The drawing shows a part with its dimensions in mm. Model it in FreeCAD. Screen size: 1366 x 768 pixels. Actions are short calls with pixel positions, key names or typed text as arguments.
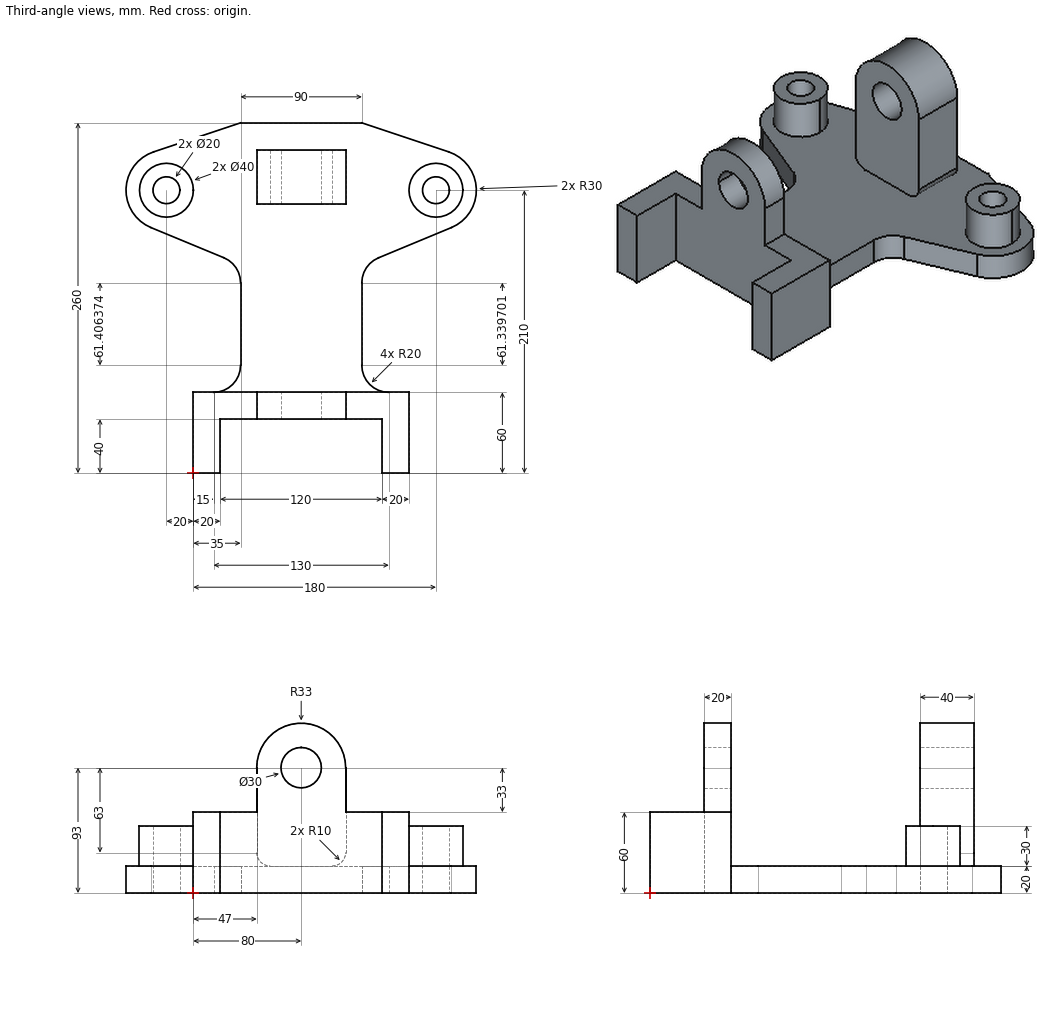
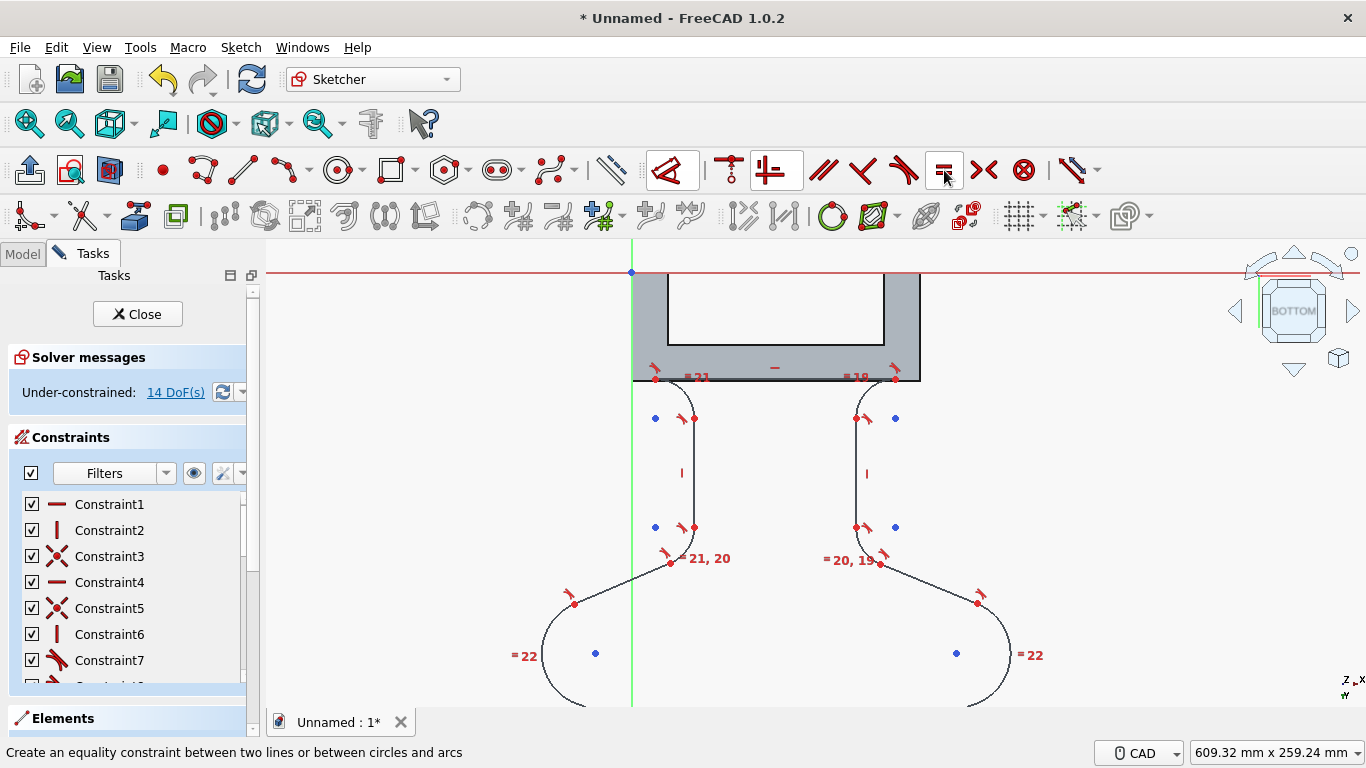
click(860, 400)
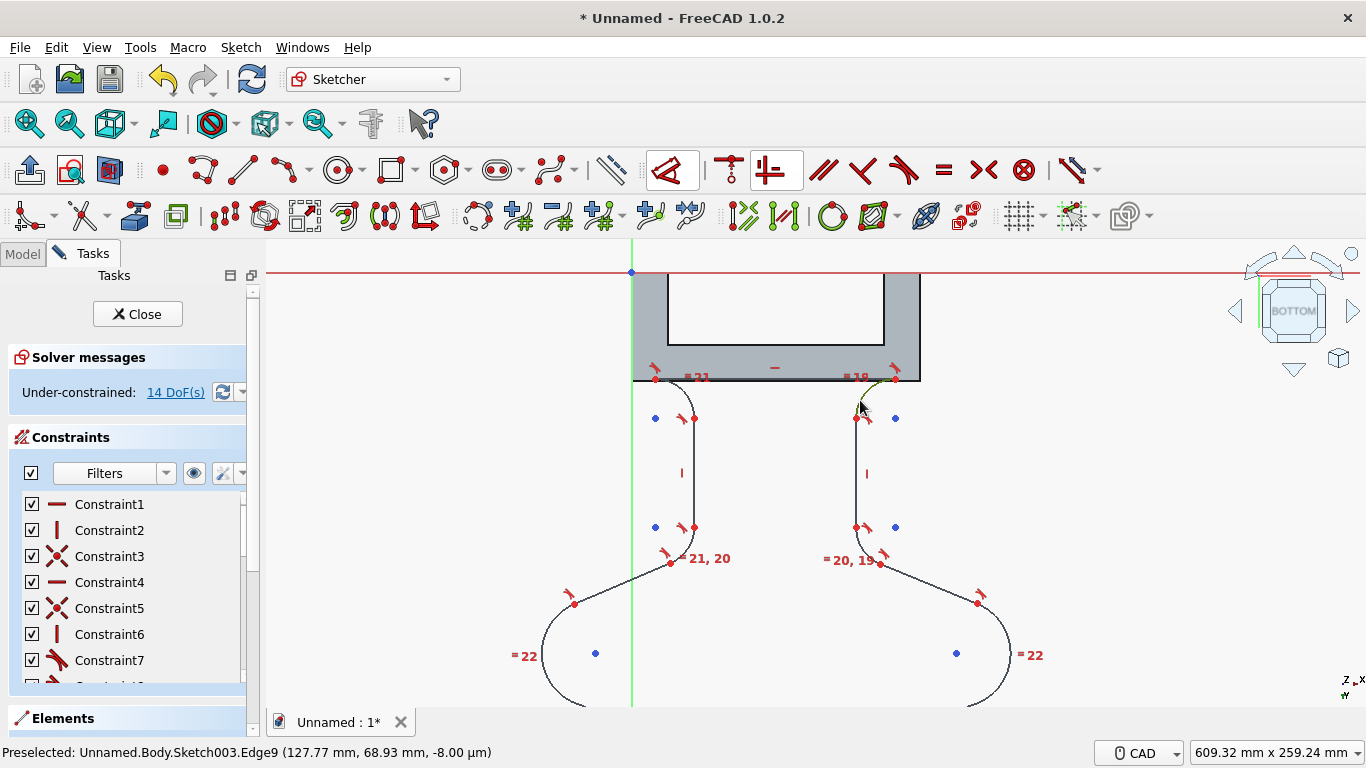
click(694, 170)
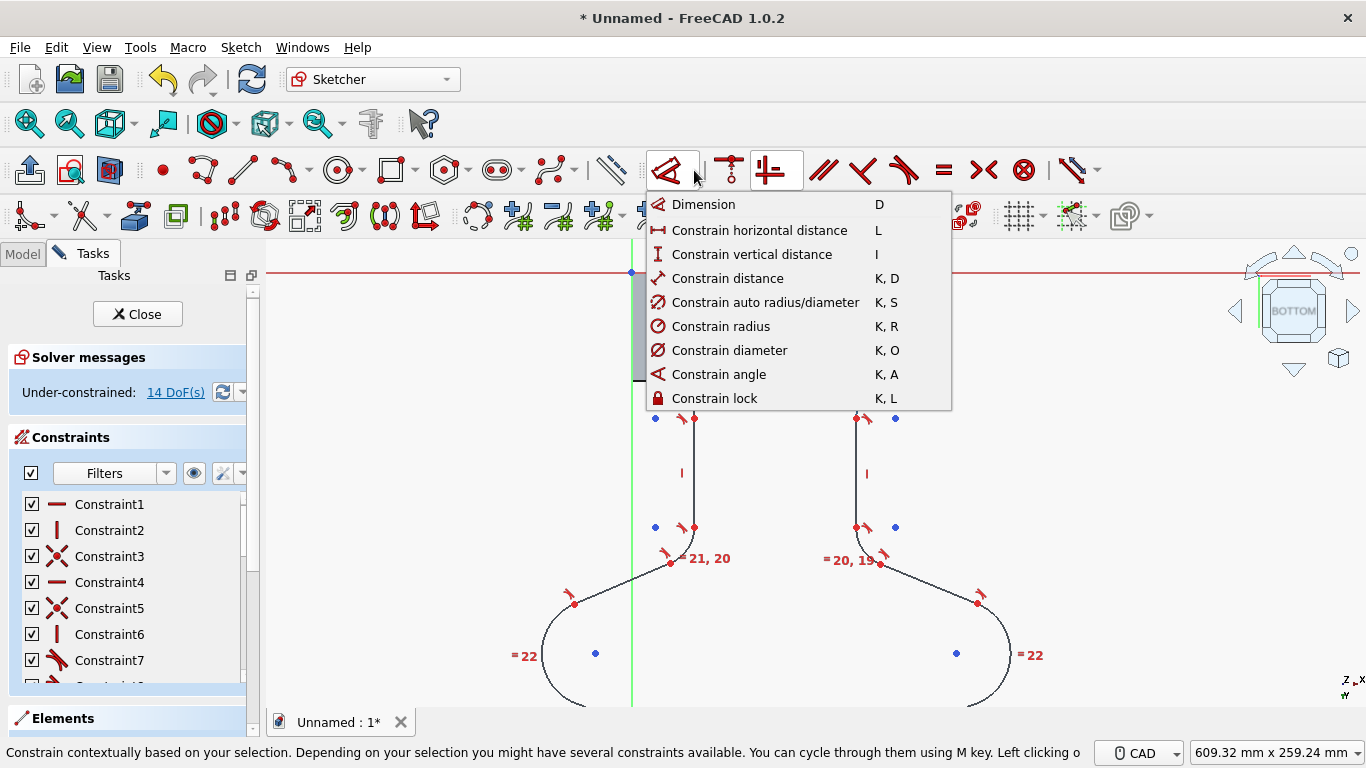
click(799, 326)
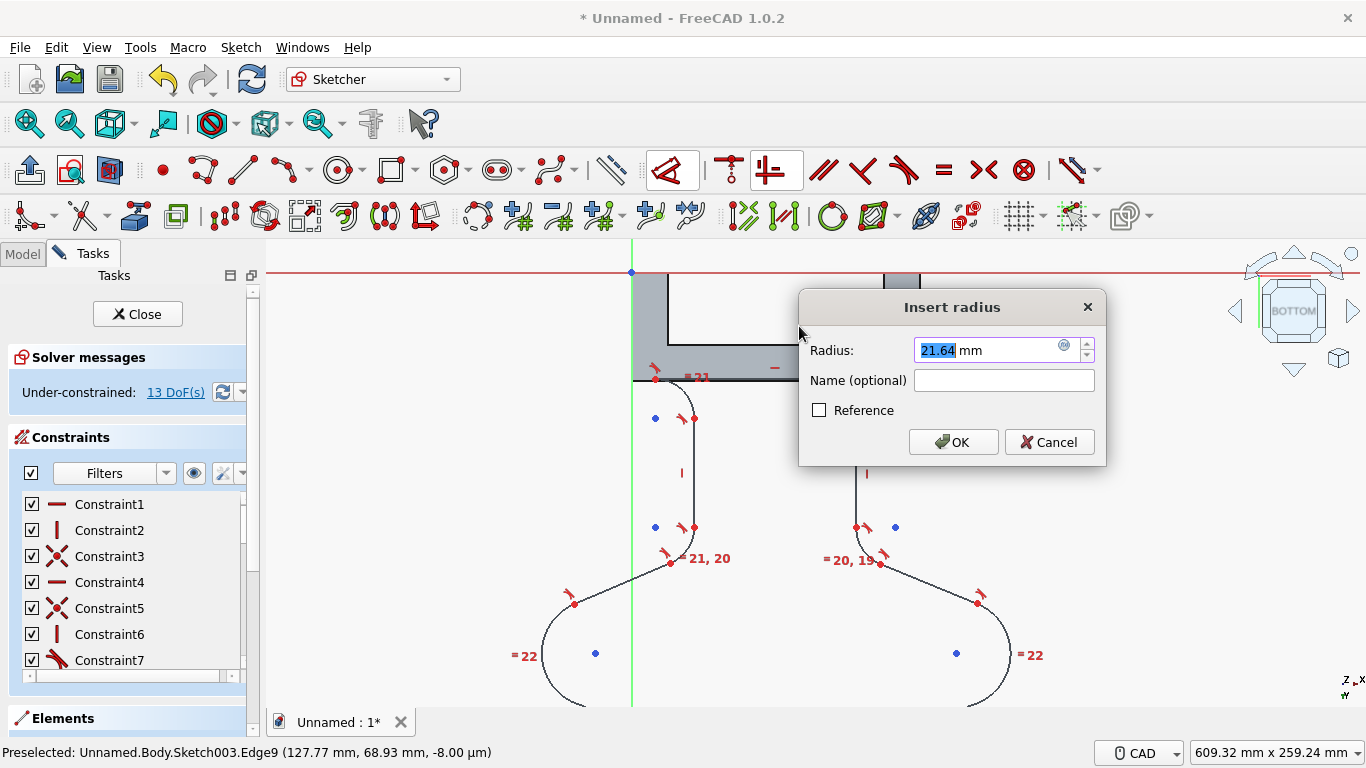
text(20)
key(Return)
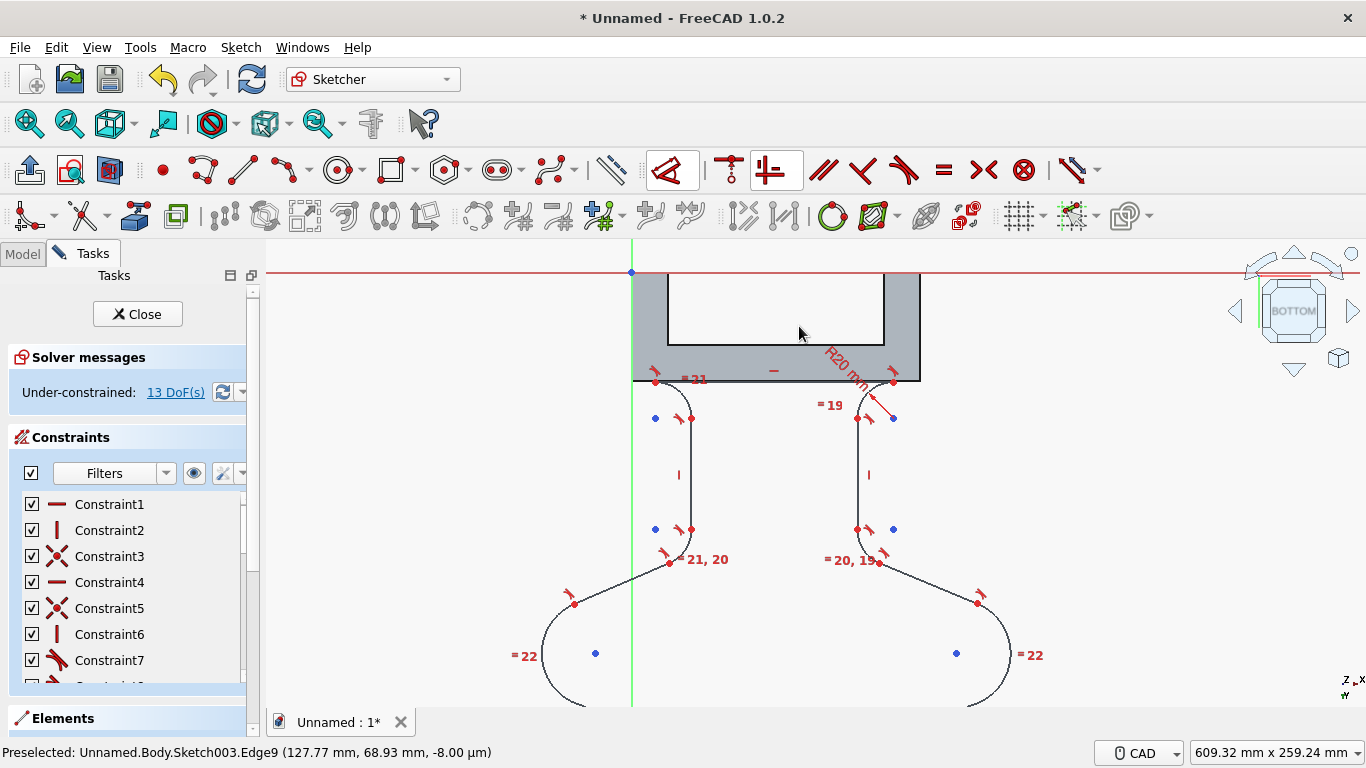
click(1005, 630)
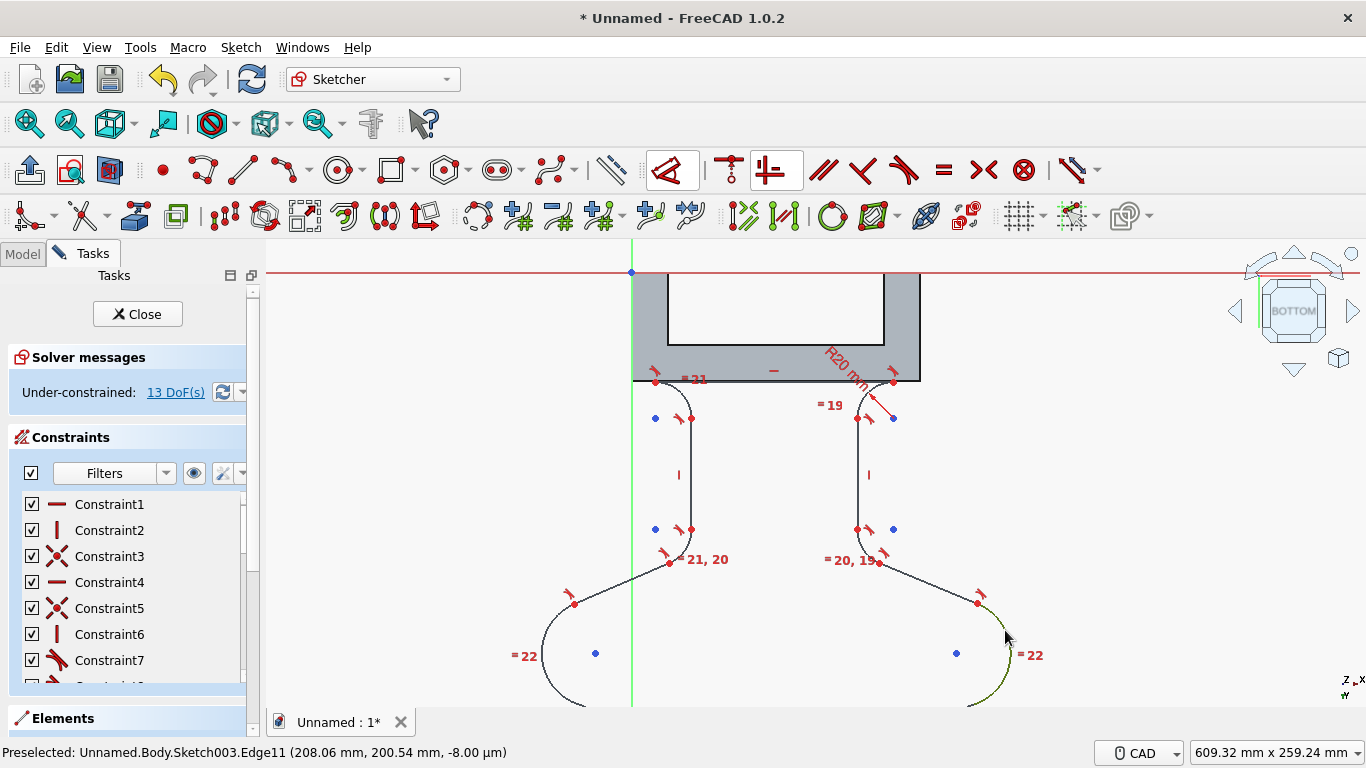
key(k)
key(r)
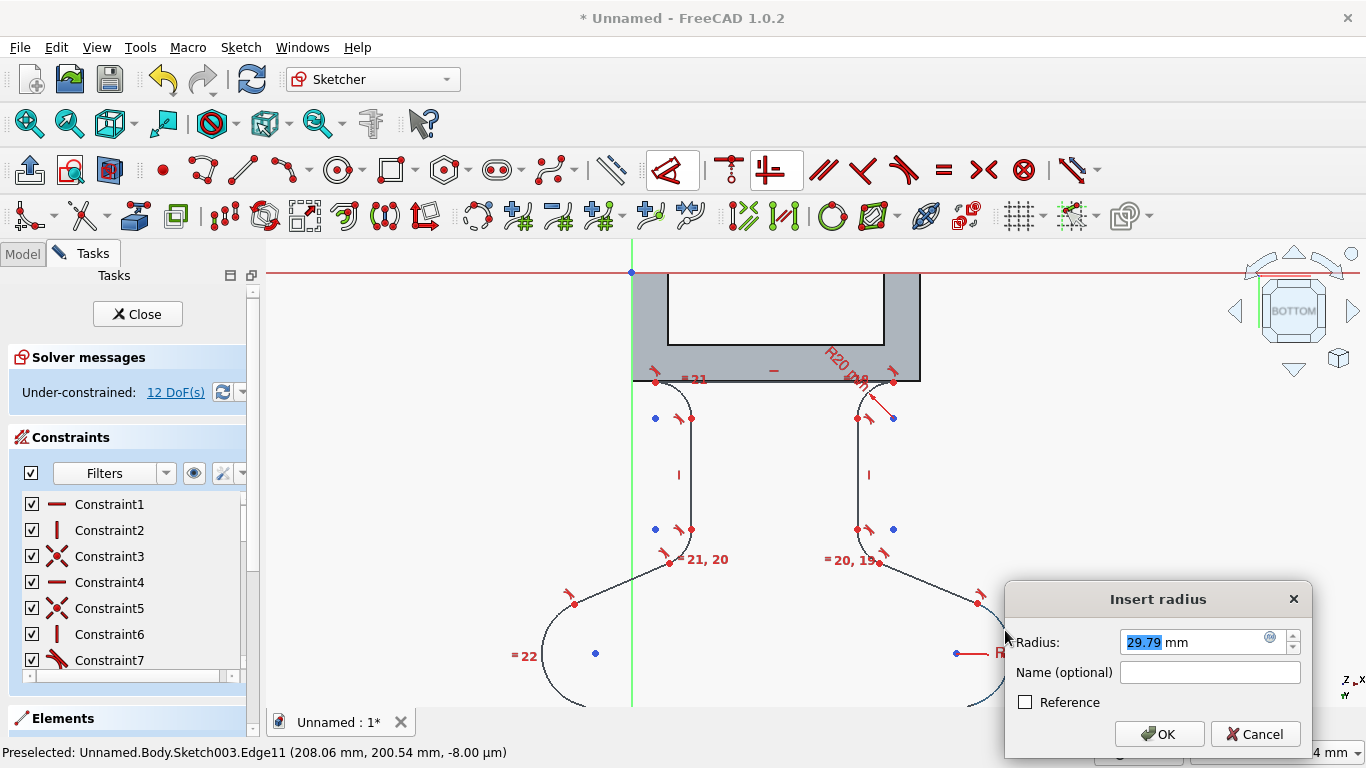
text(30)
key(Return)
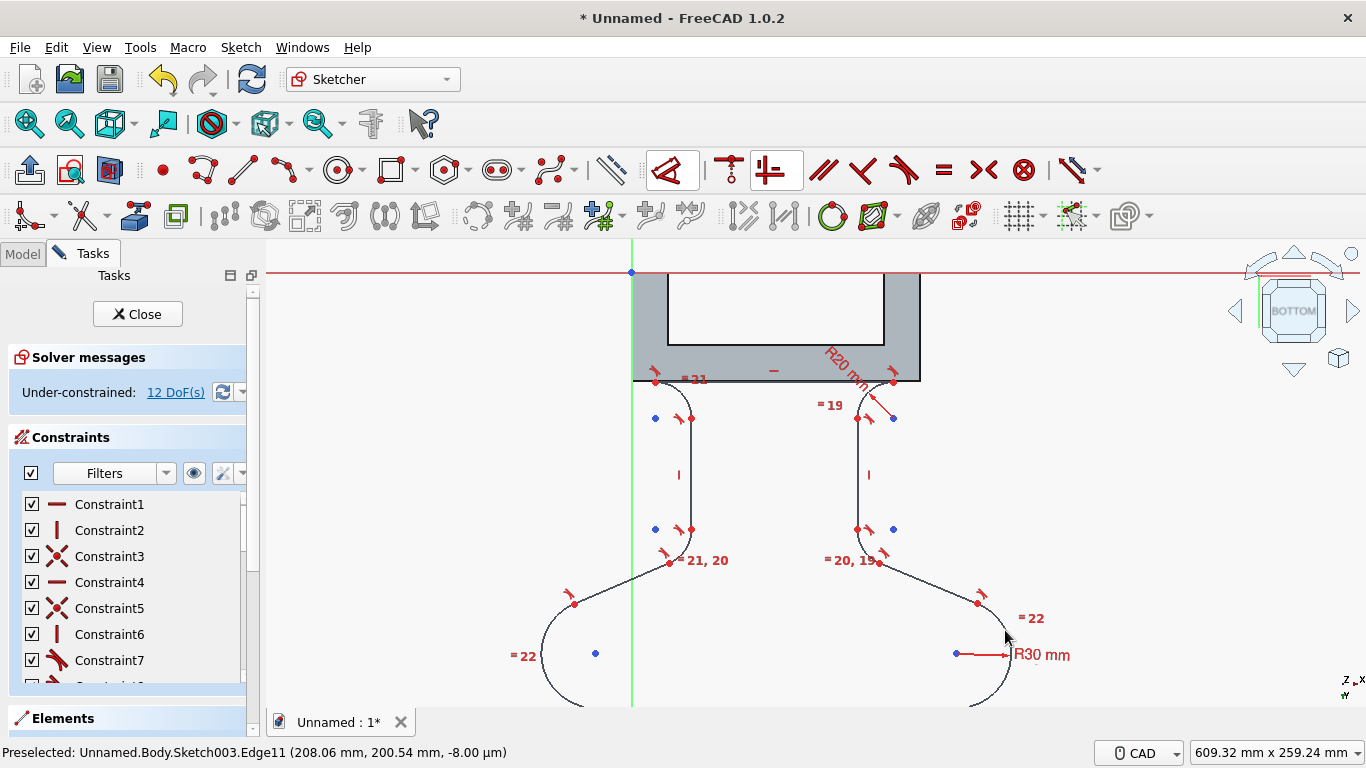
scroll(689, 403, down, 2)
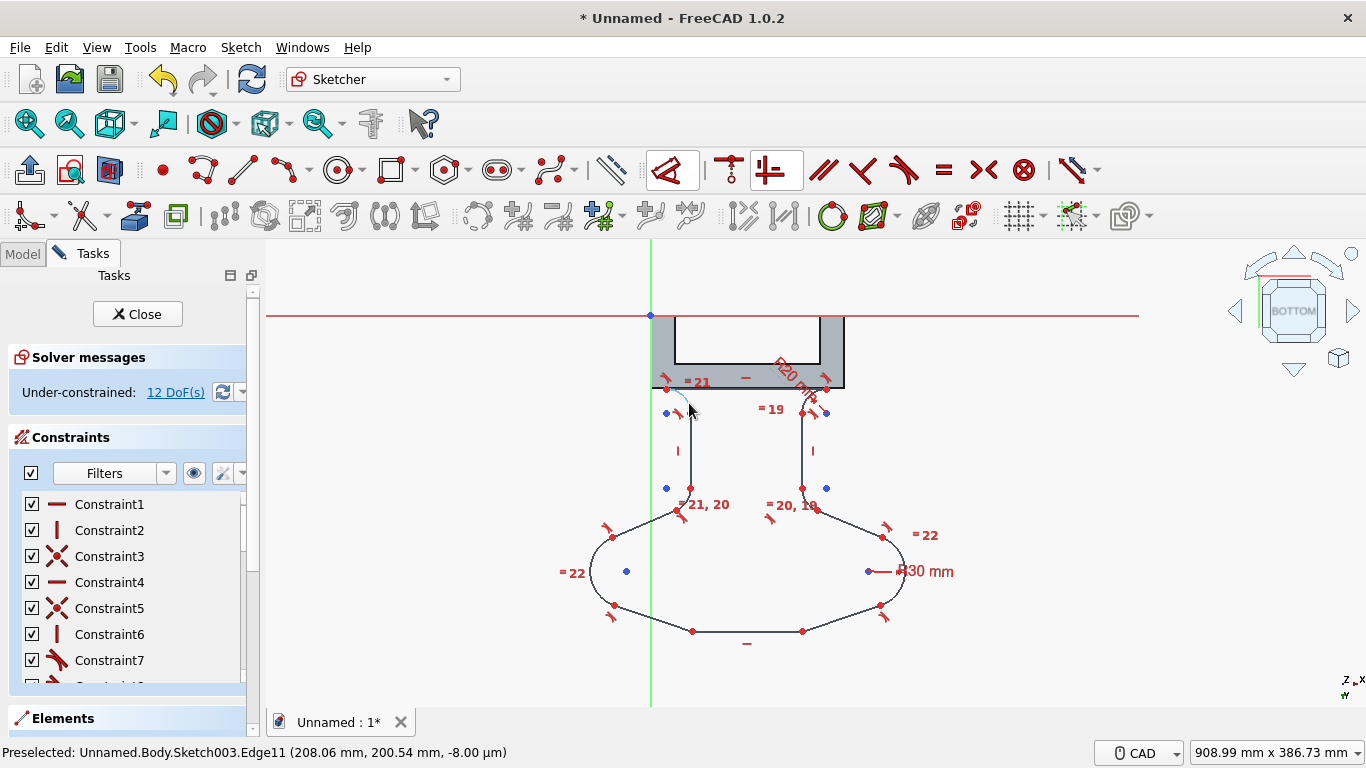
click(770, 632)